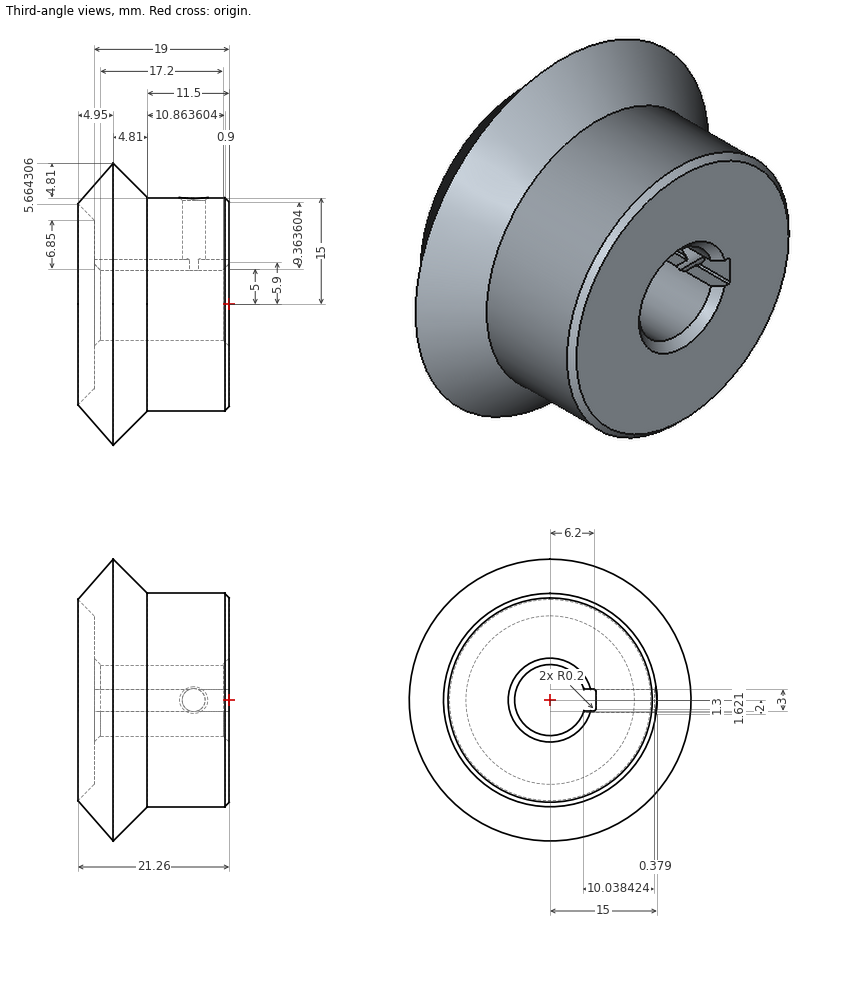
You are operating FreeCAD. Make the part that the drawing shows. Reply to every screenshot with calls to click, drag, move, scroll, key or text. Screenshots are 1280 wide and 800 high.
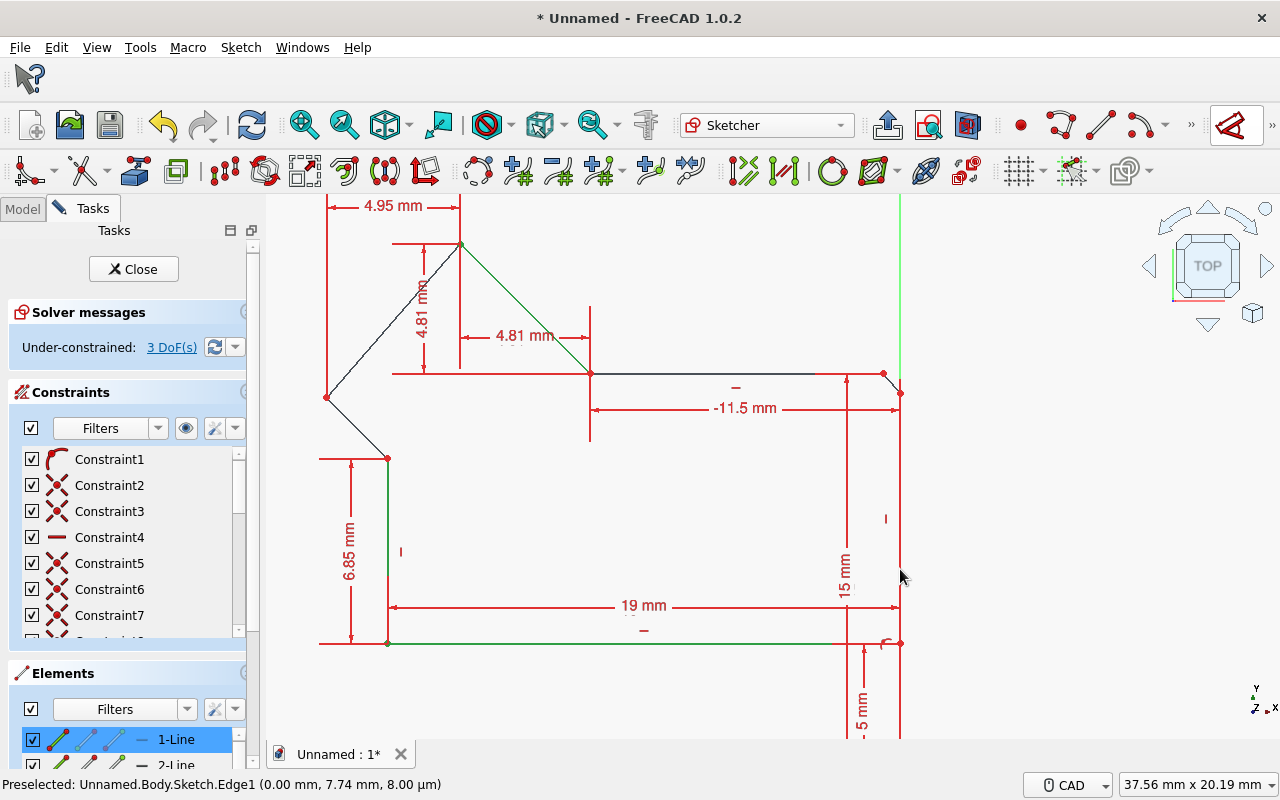
click(1258, 126)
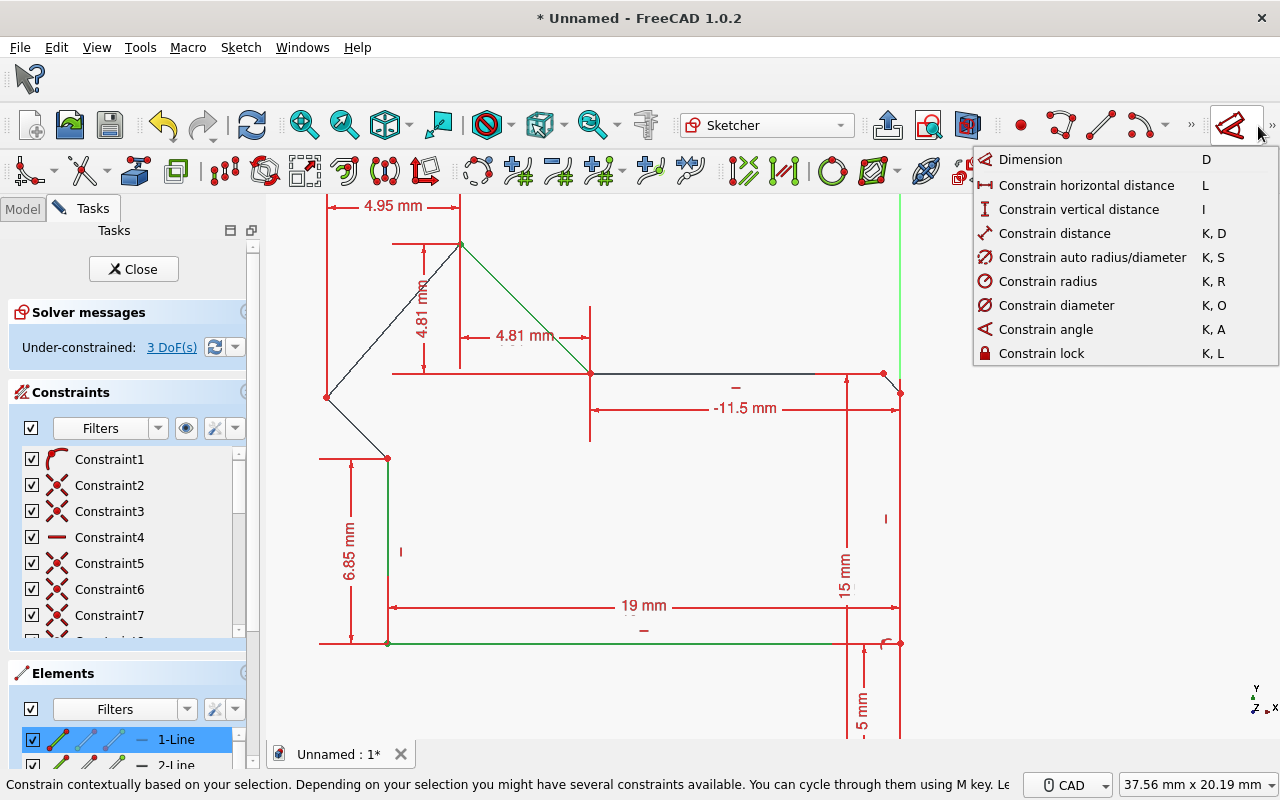
click(1126, 209)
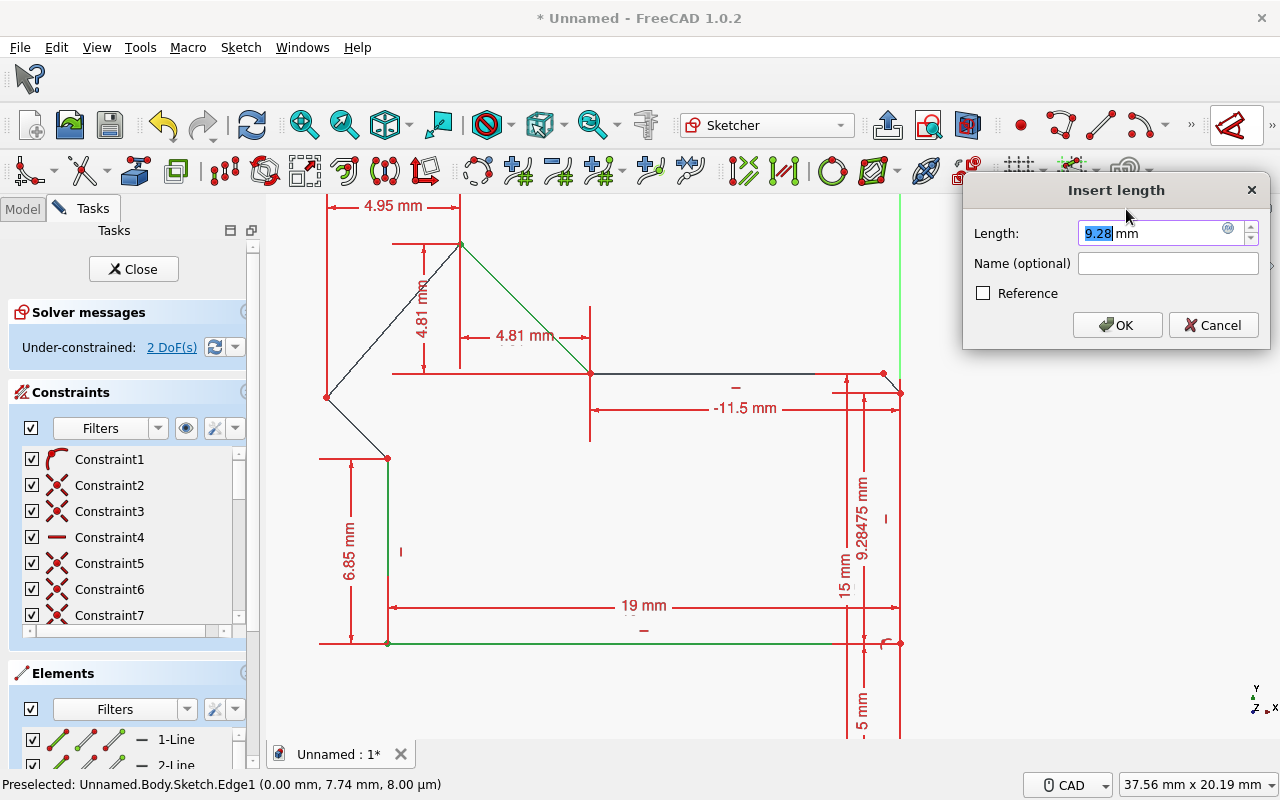
text(9.363604)
key(Return)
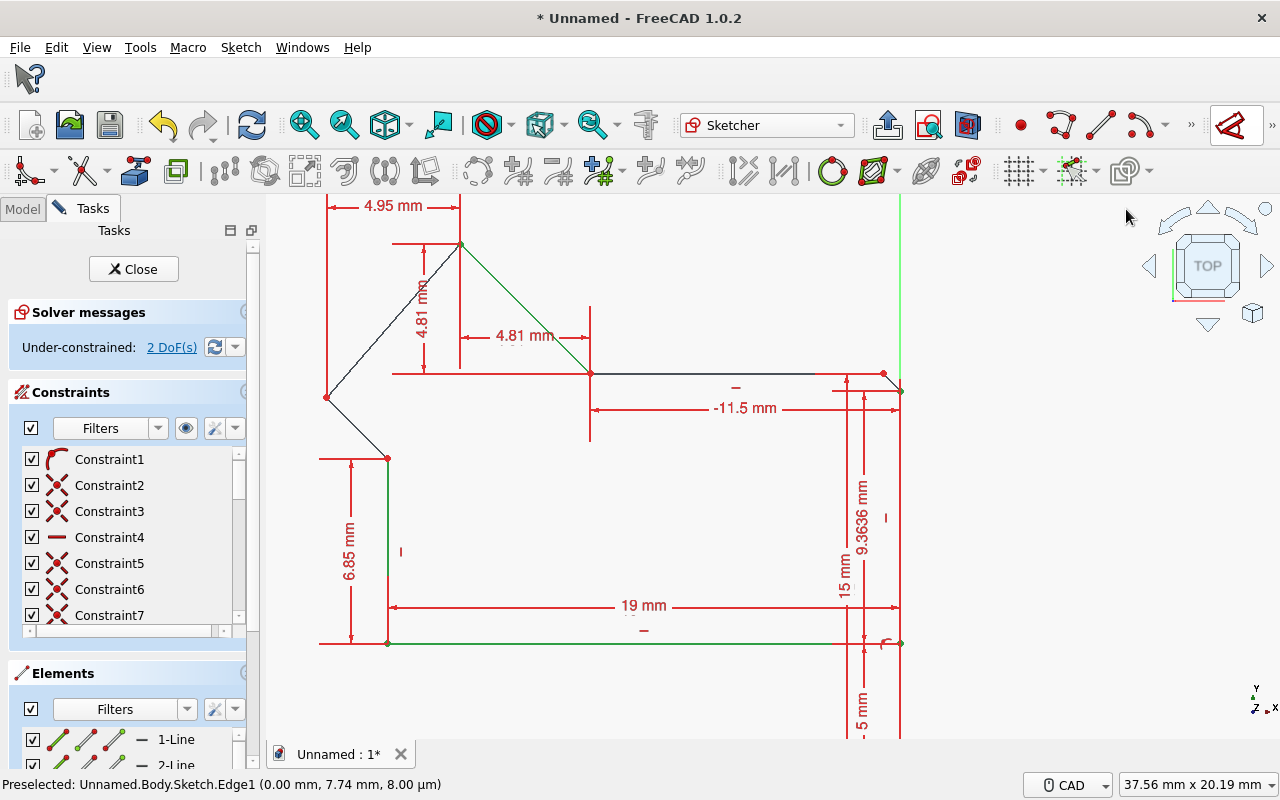
click(795, 374)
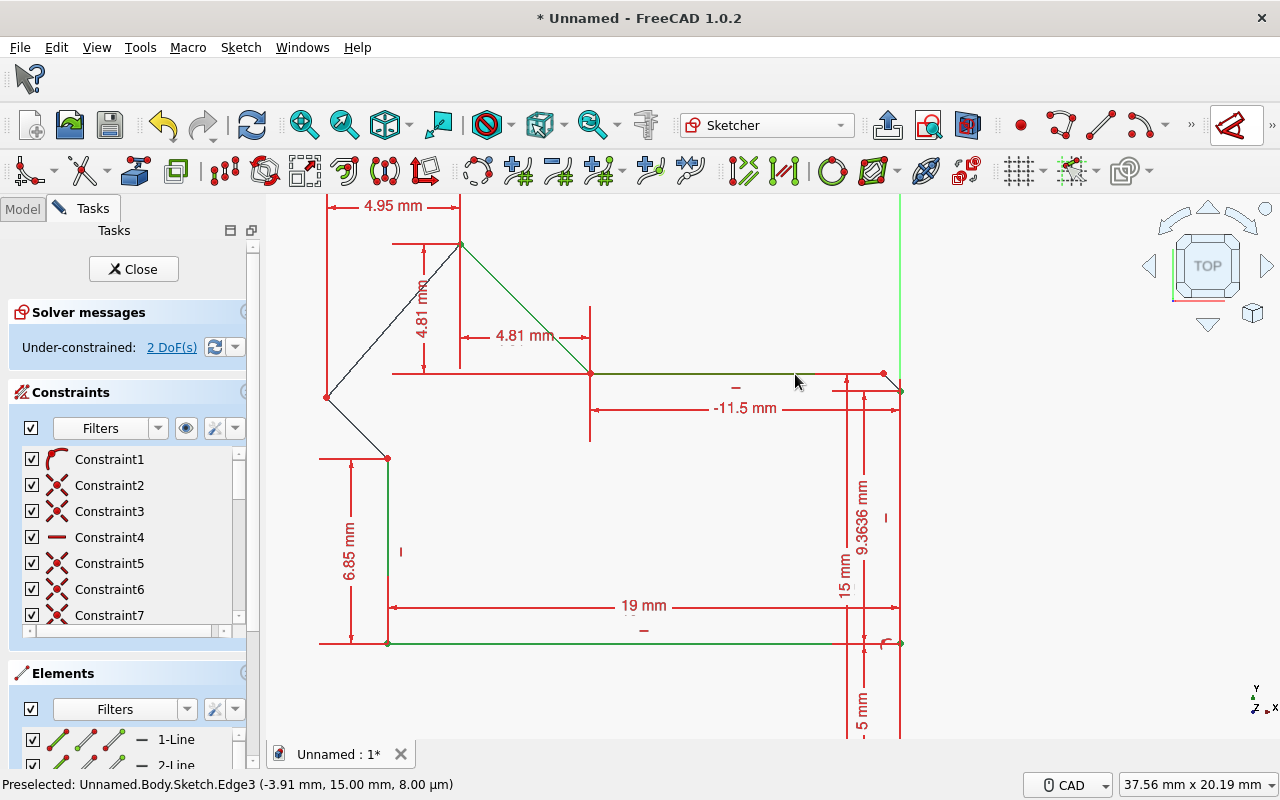
key(l)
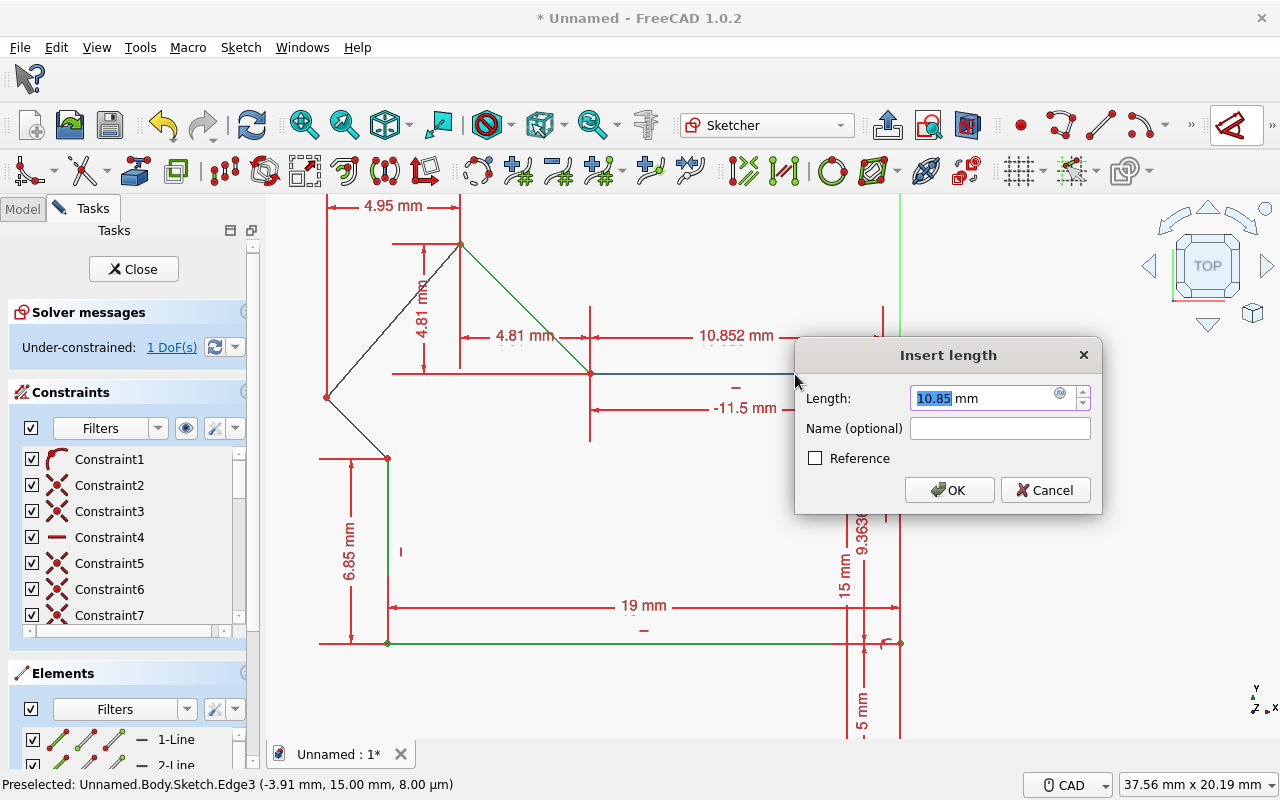
text(10.863604)
key(Return)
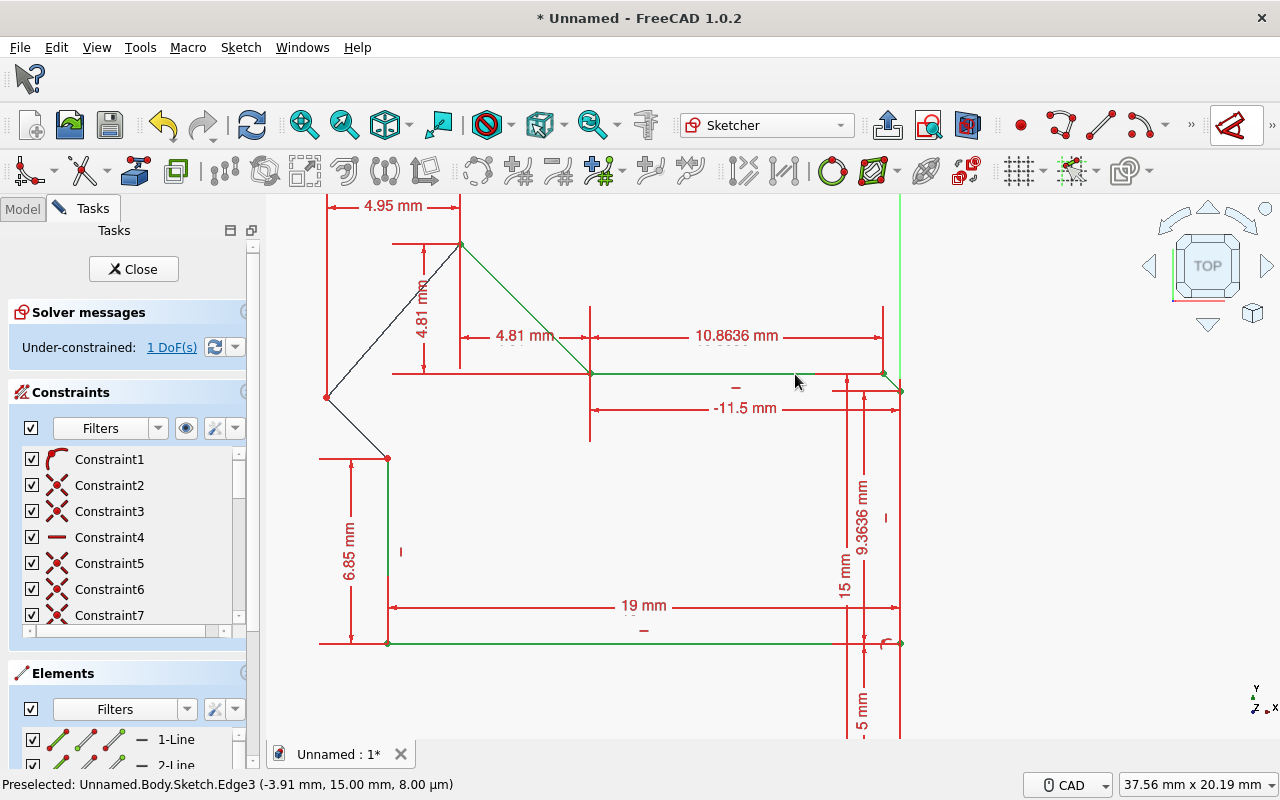
click(367, 352)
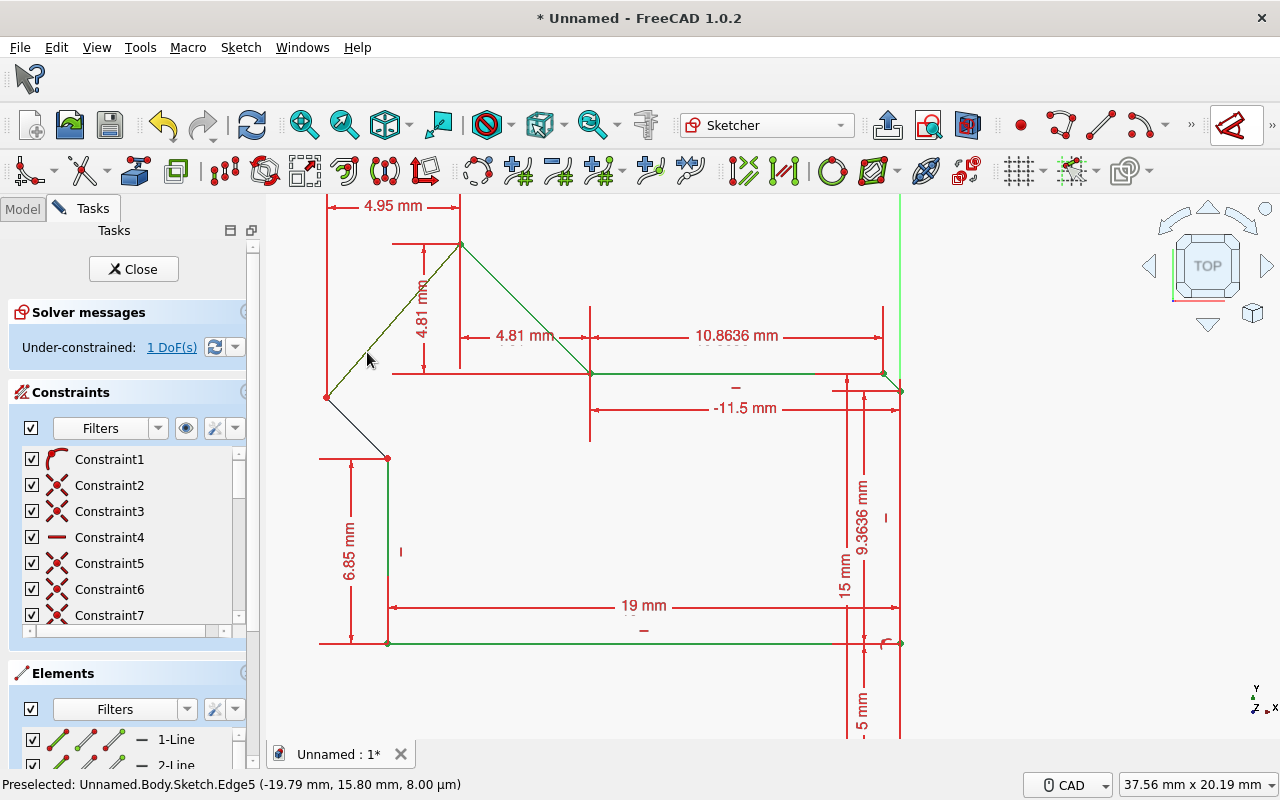
click(1258, 126)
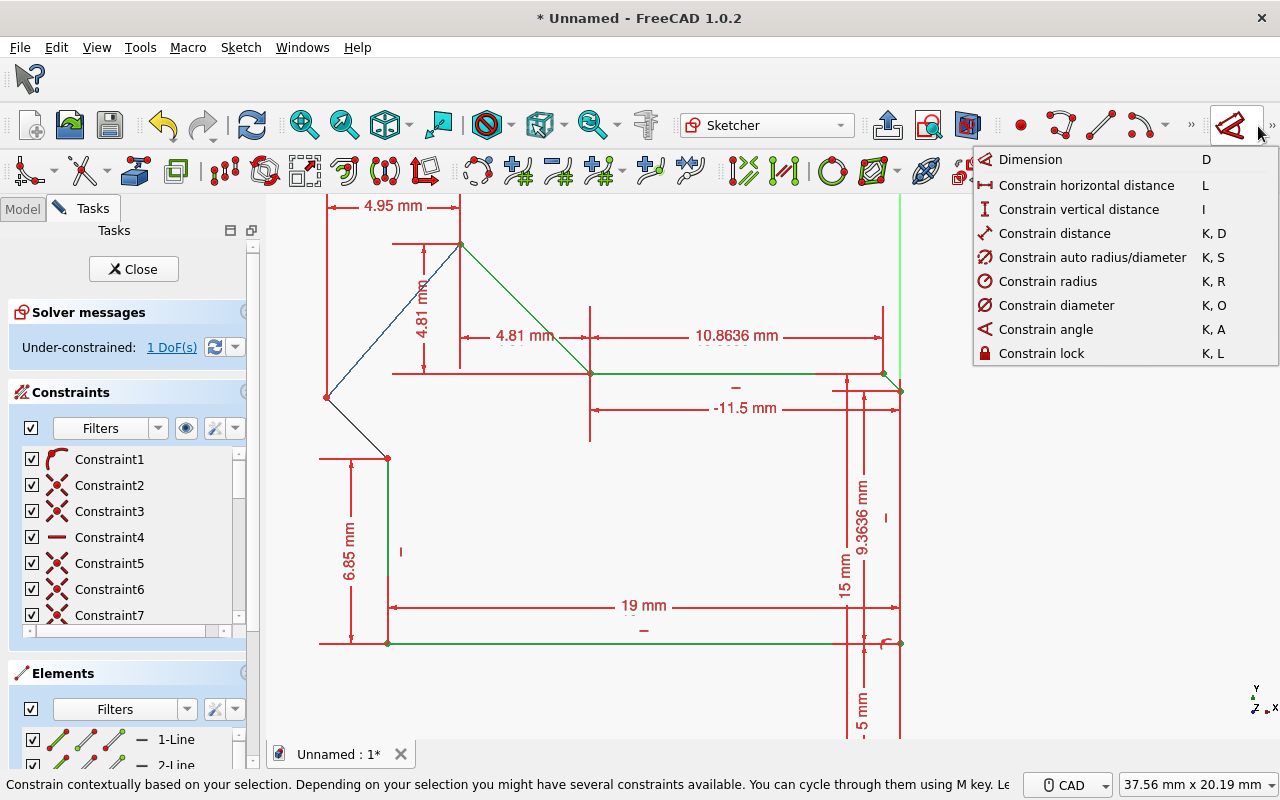
click(1126, 209)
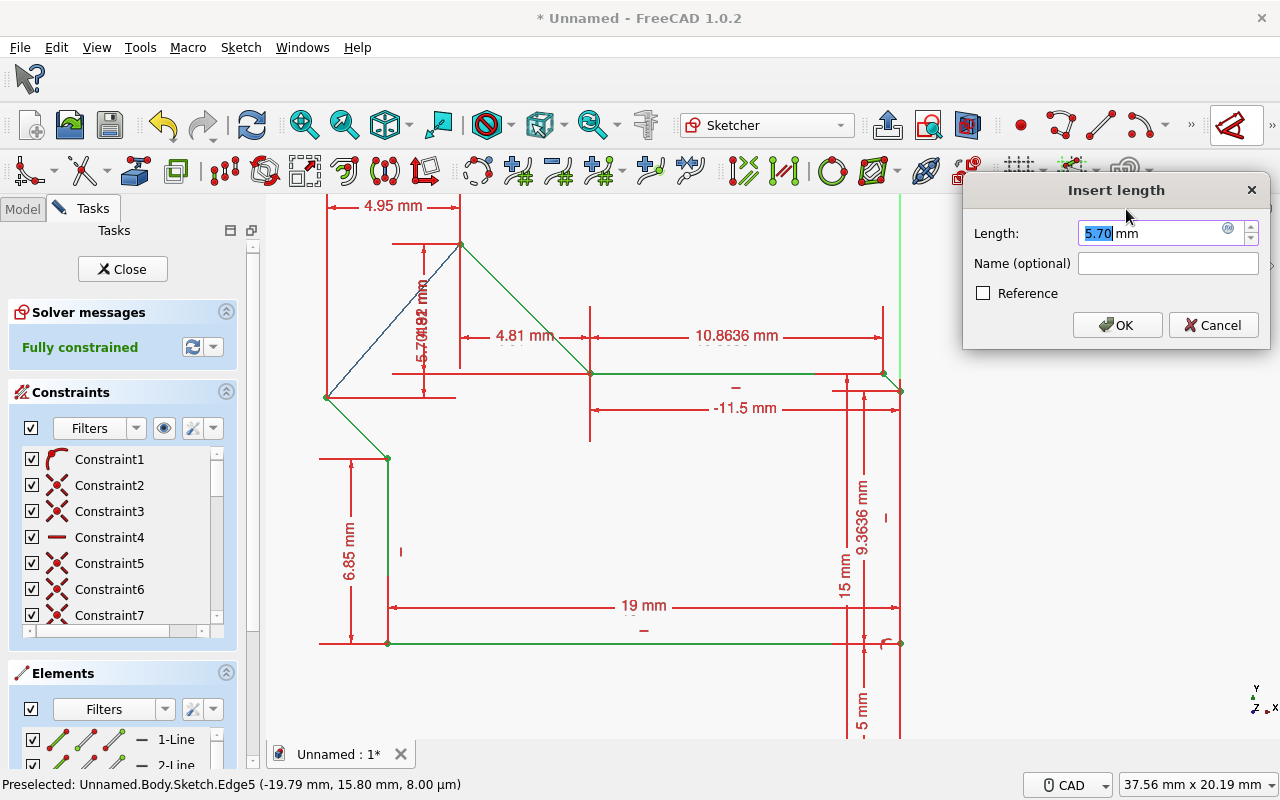
text(5.664306)
key(Return)